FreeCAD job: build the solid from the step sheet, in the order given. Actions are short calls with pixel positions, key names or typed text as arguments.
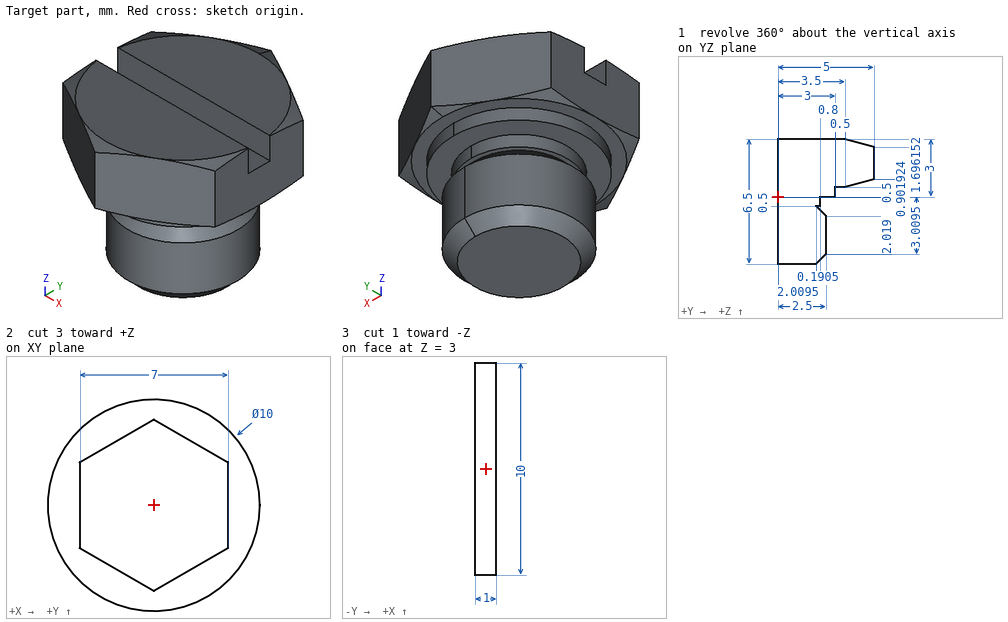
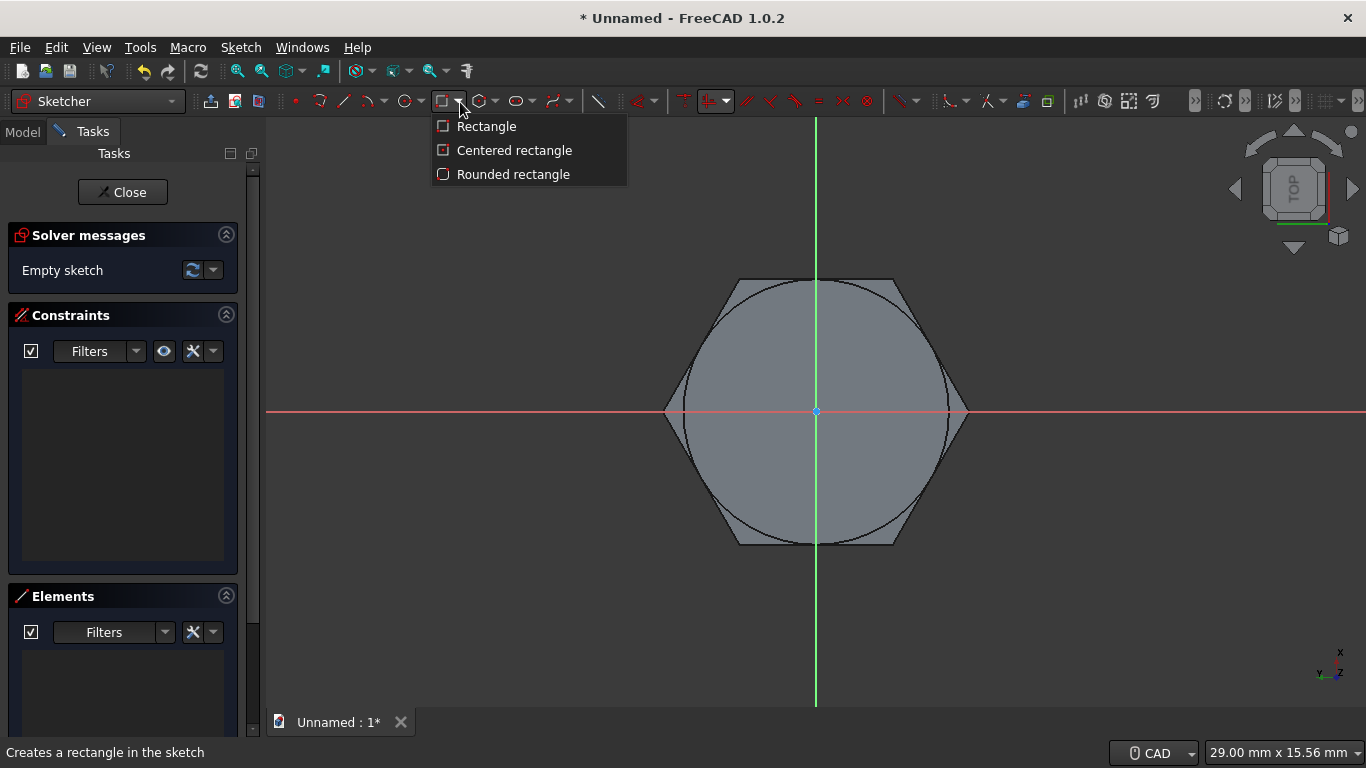
click(530, 150)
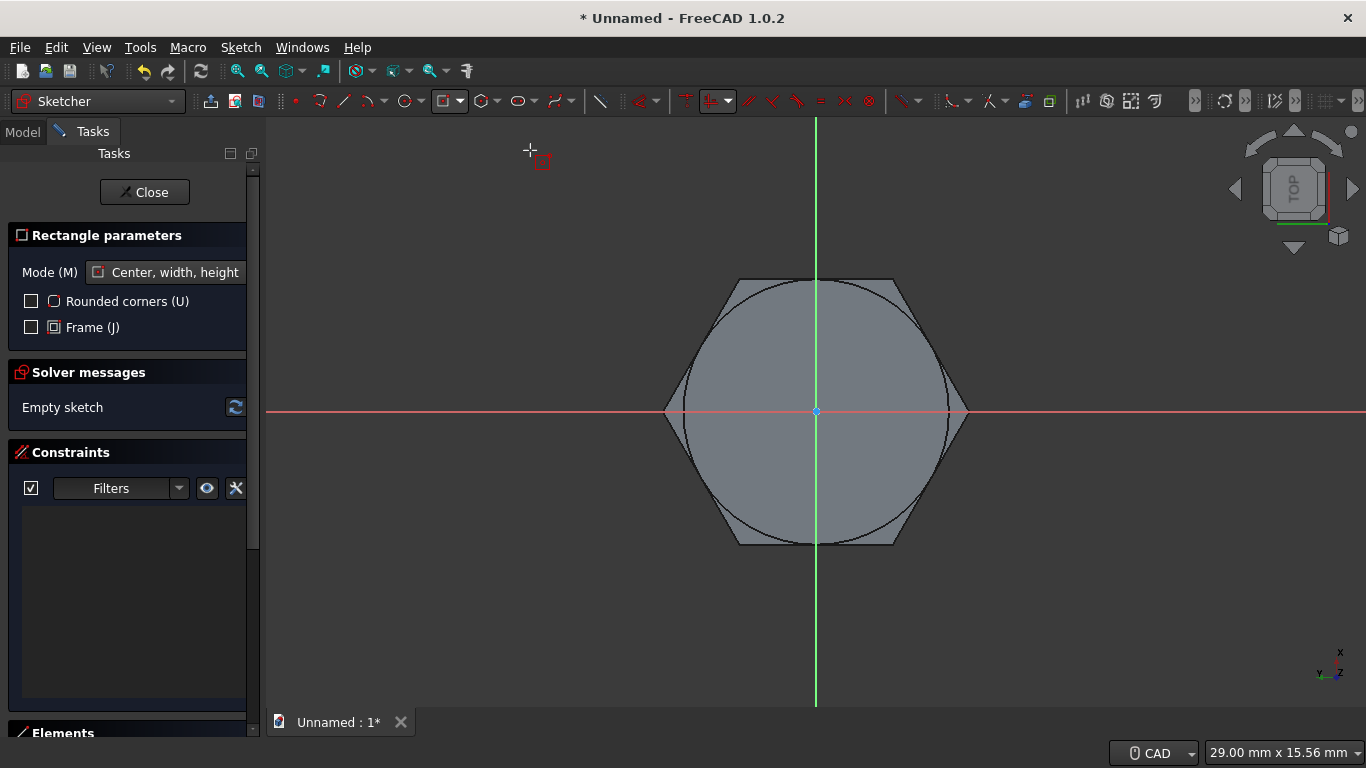
click(816, 412)
click(835, 222)
key(Escape)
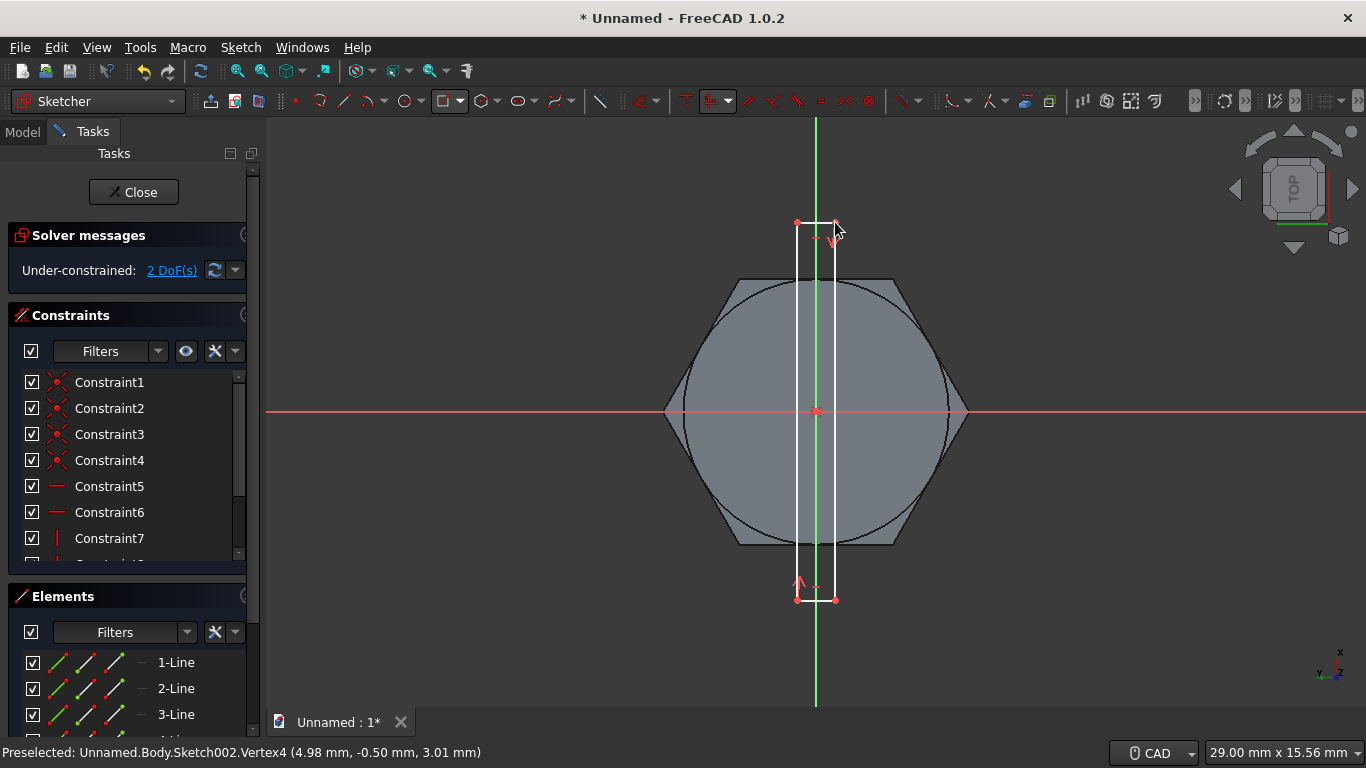
key(d)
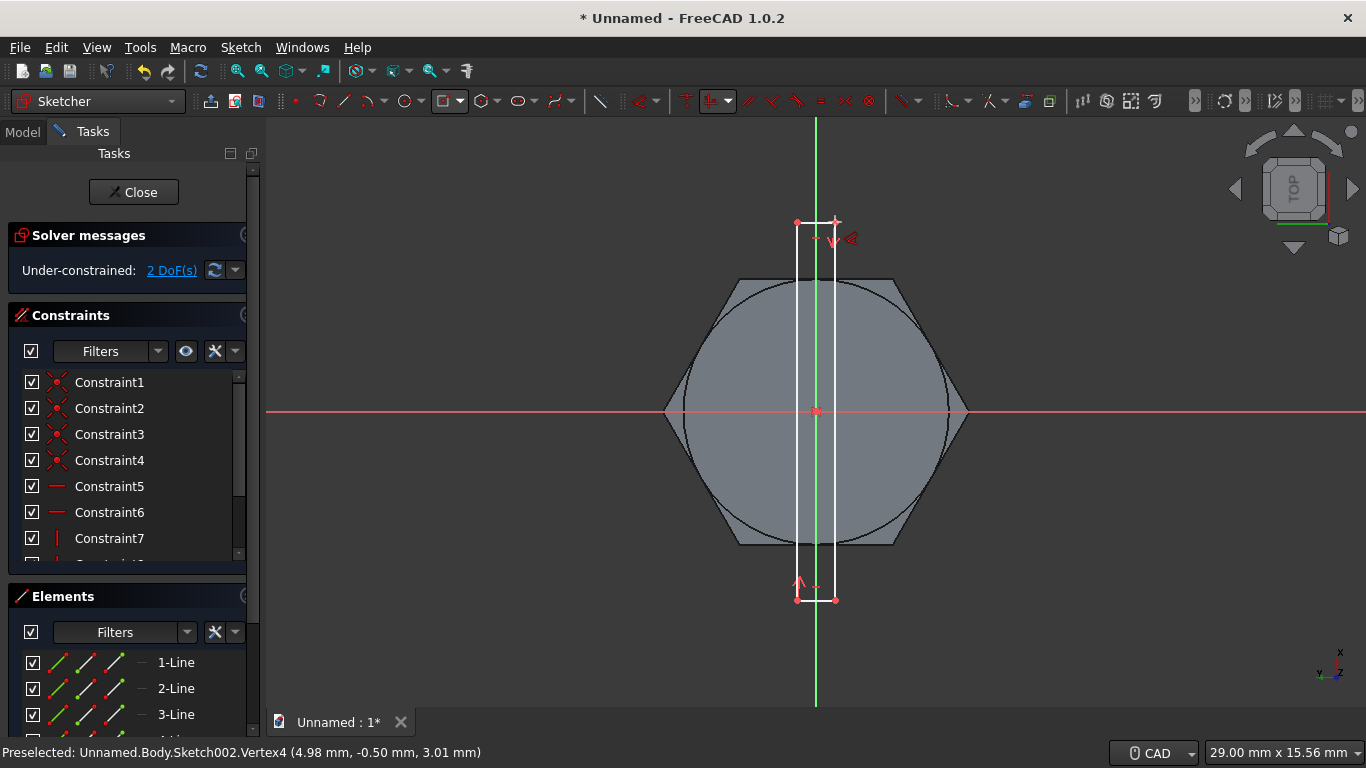
click(812, 601)
click(803, 635)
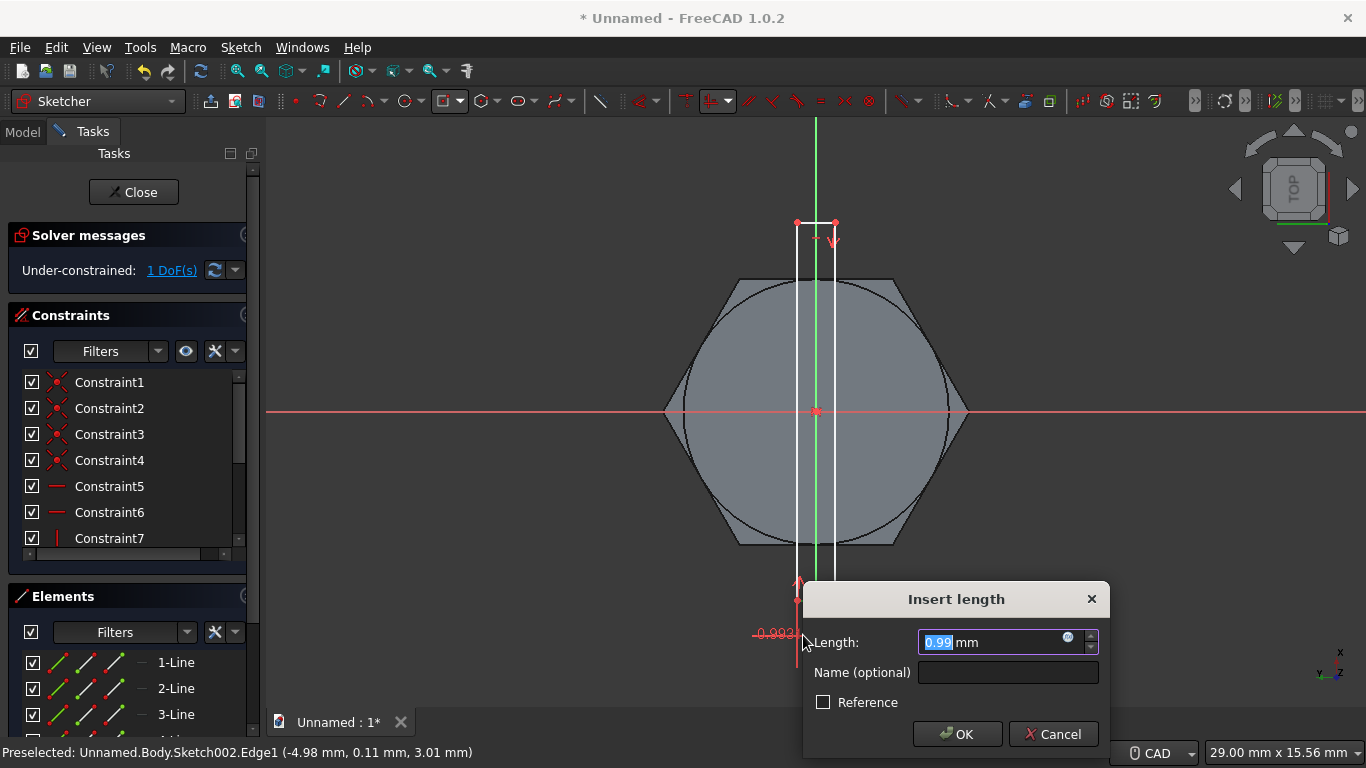
text(1)
key(Return)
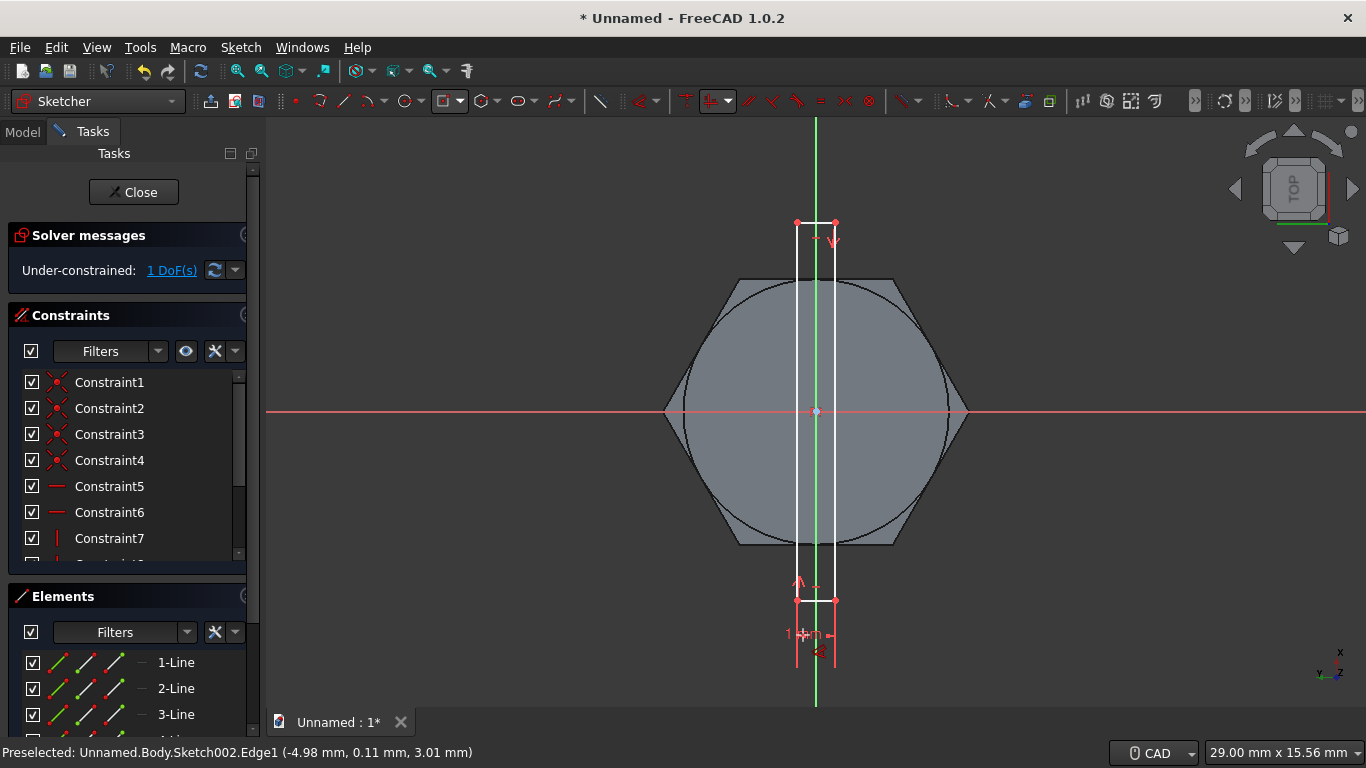
click(835, 488)
click(869, 325)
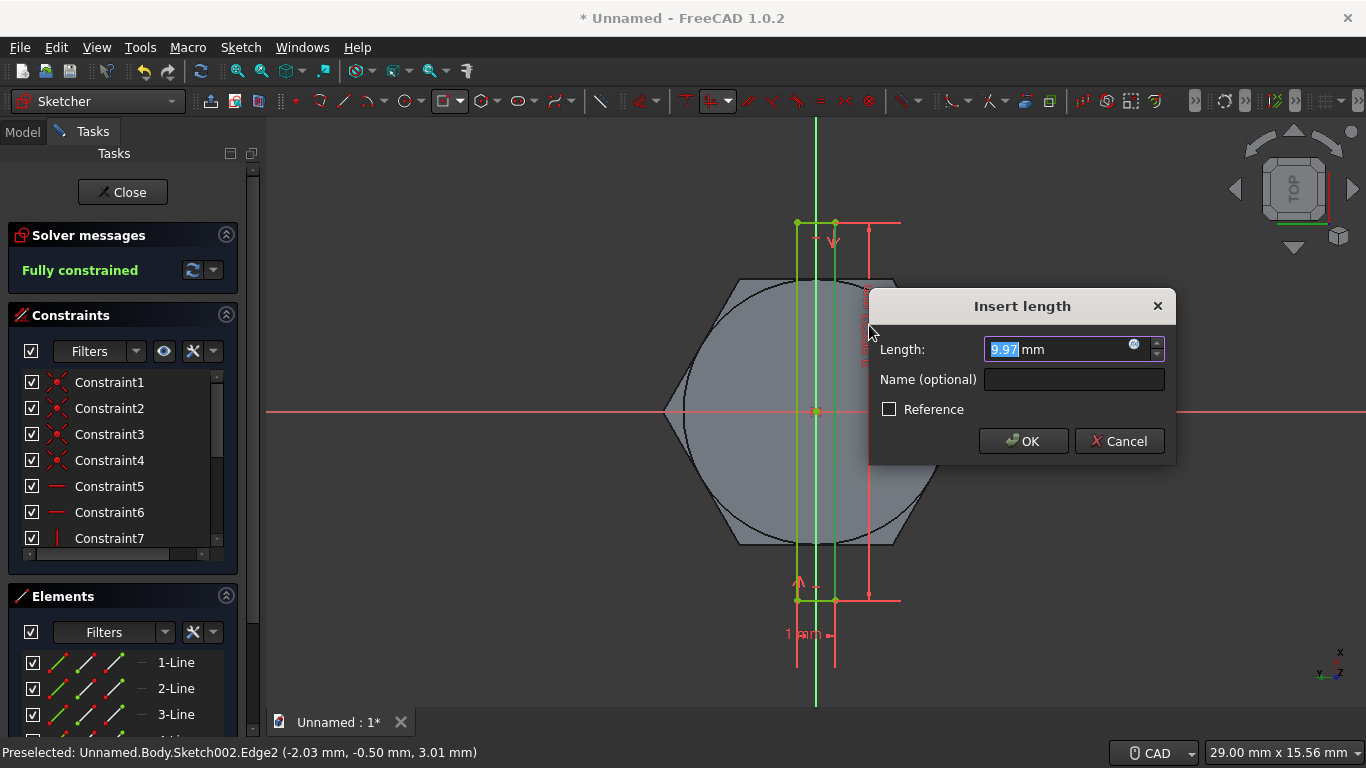
text(10)
key(Return)
key(Escape)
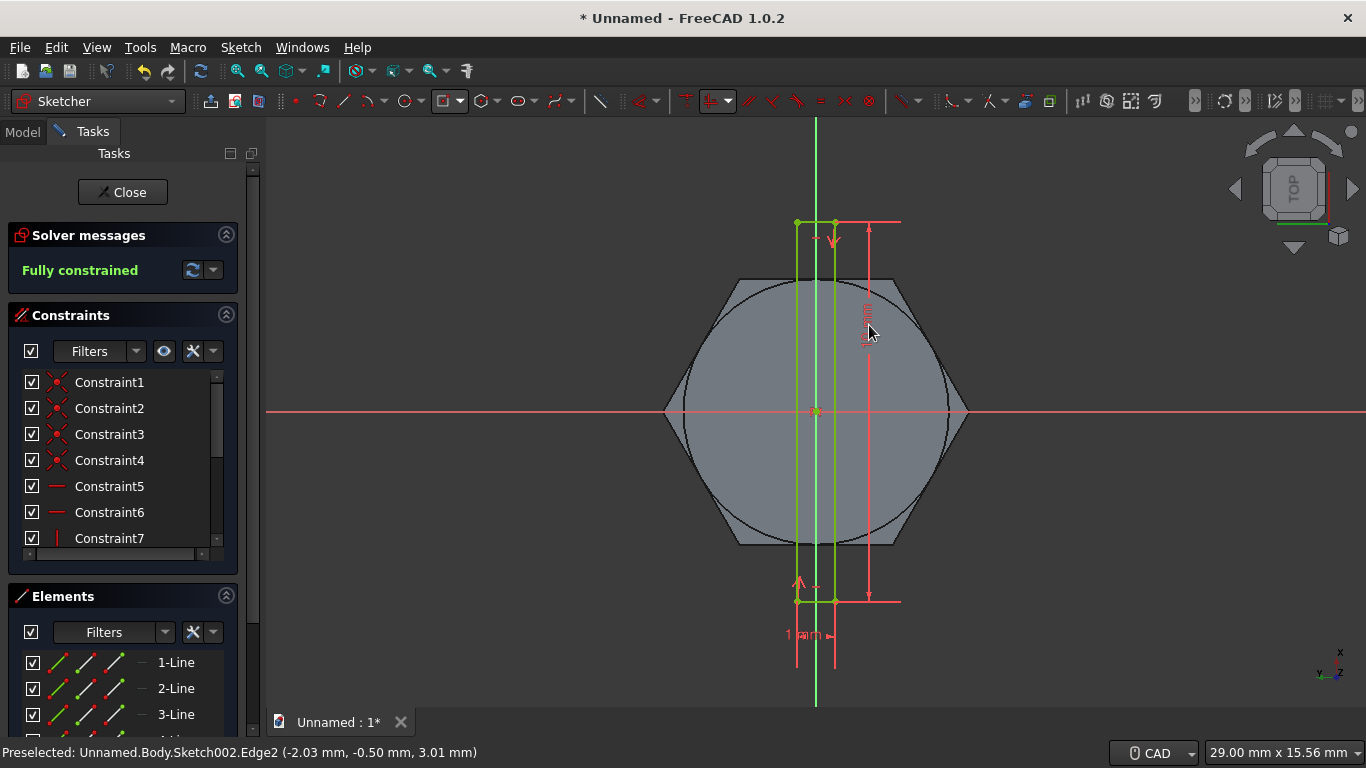
click(123, 192)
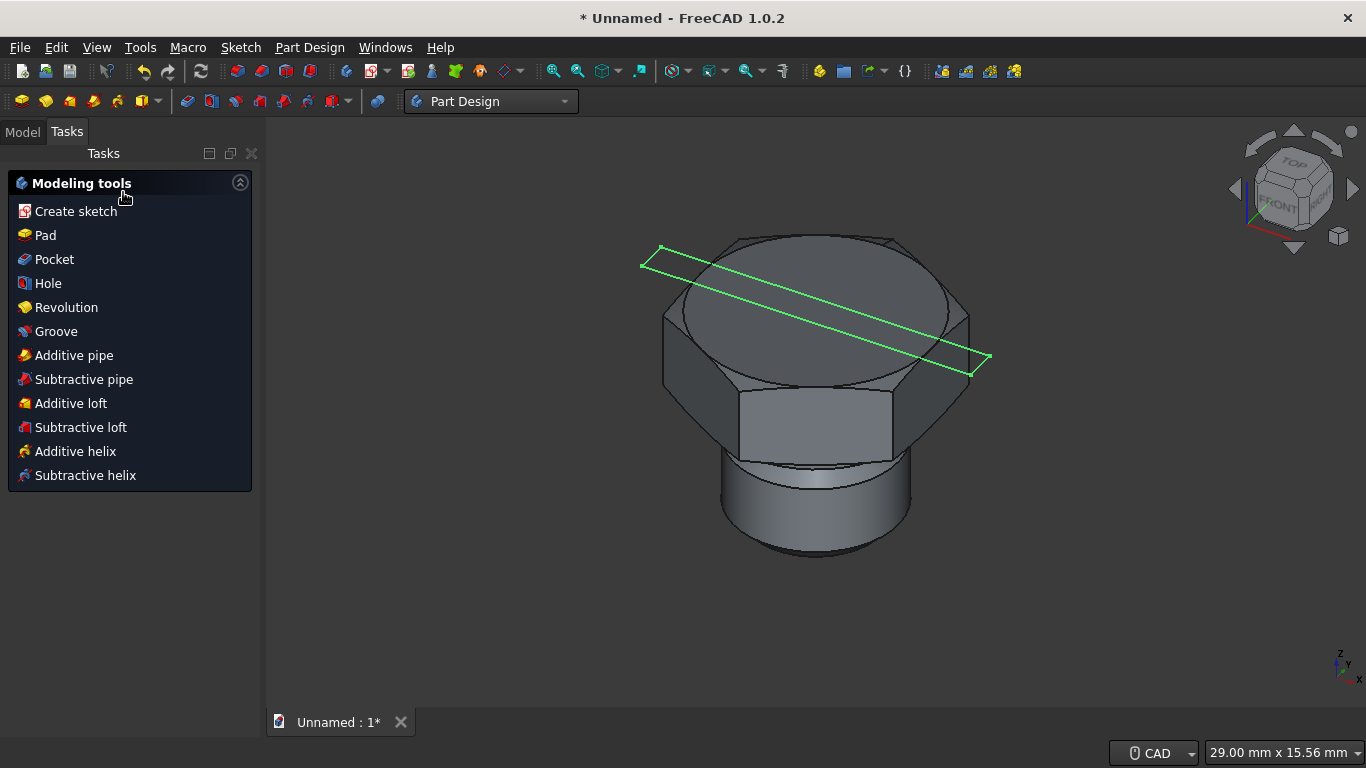
click(188, 102)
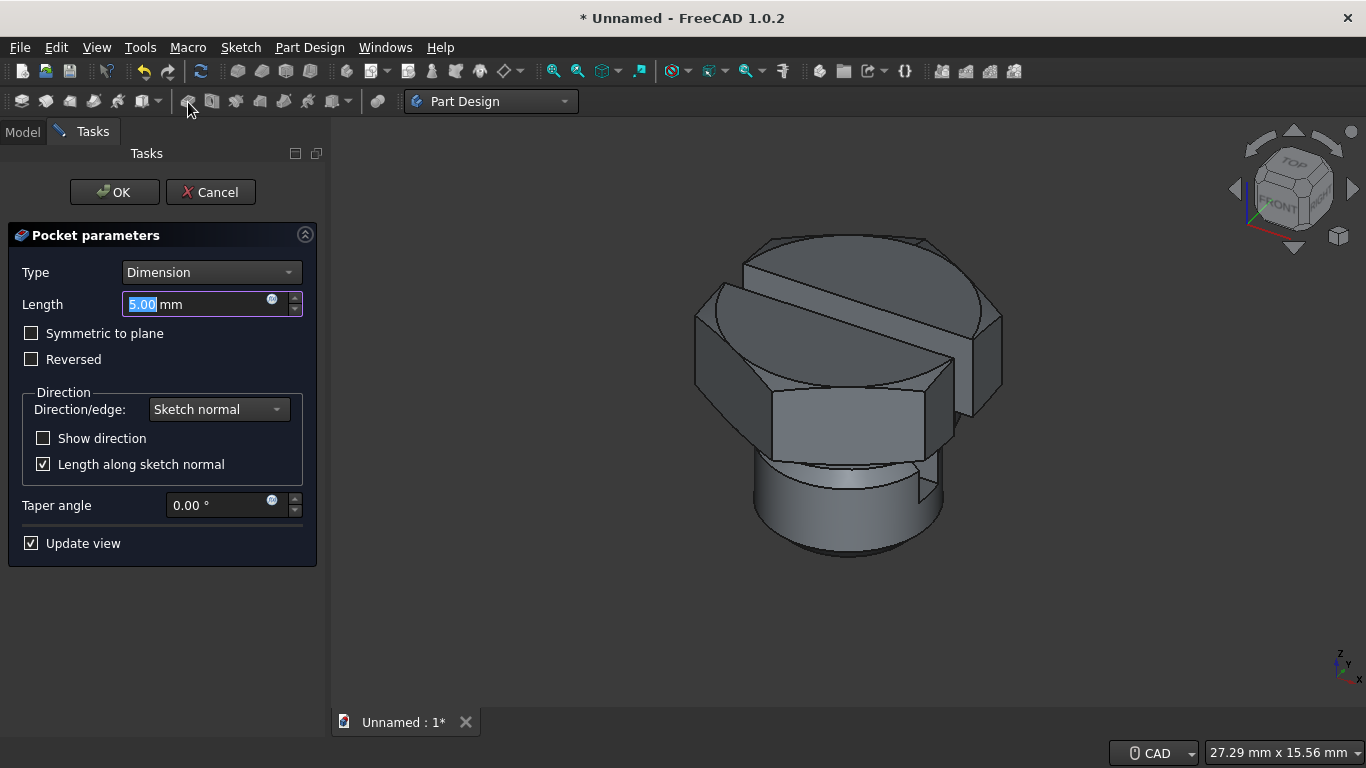
text(1)
key(Tab)